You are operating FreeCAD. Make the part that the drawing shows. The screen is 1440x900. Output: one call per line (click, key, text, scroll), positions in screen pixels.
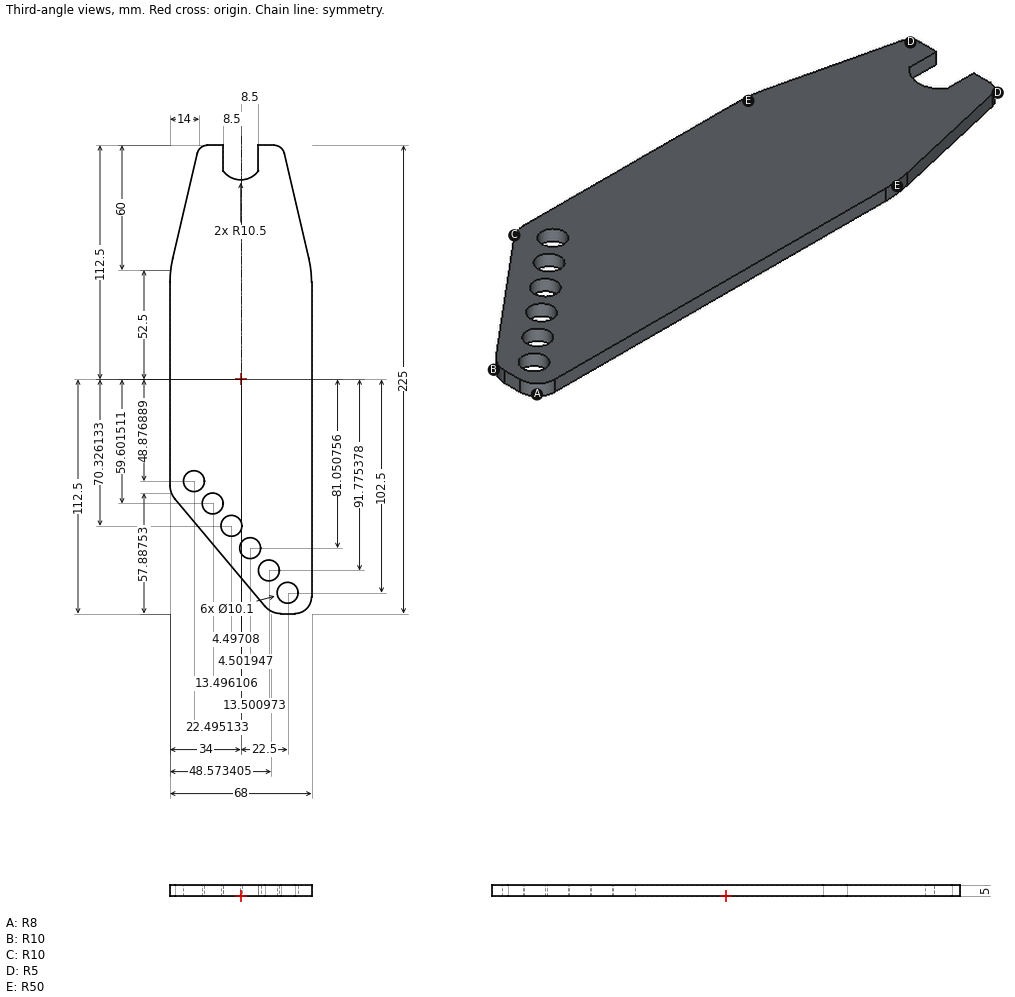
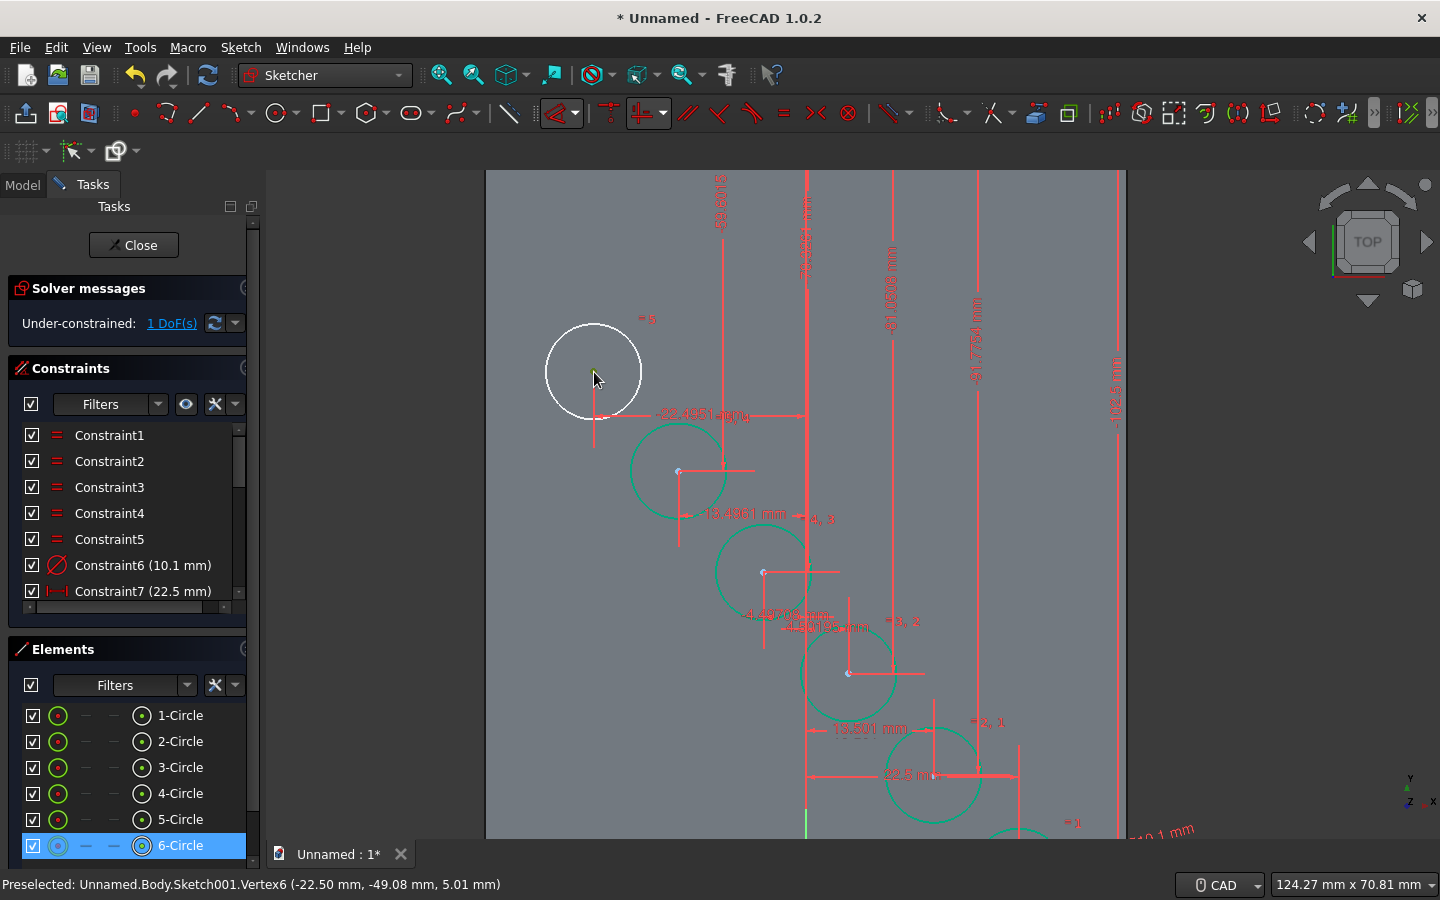
key(i)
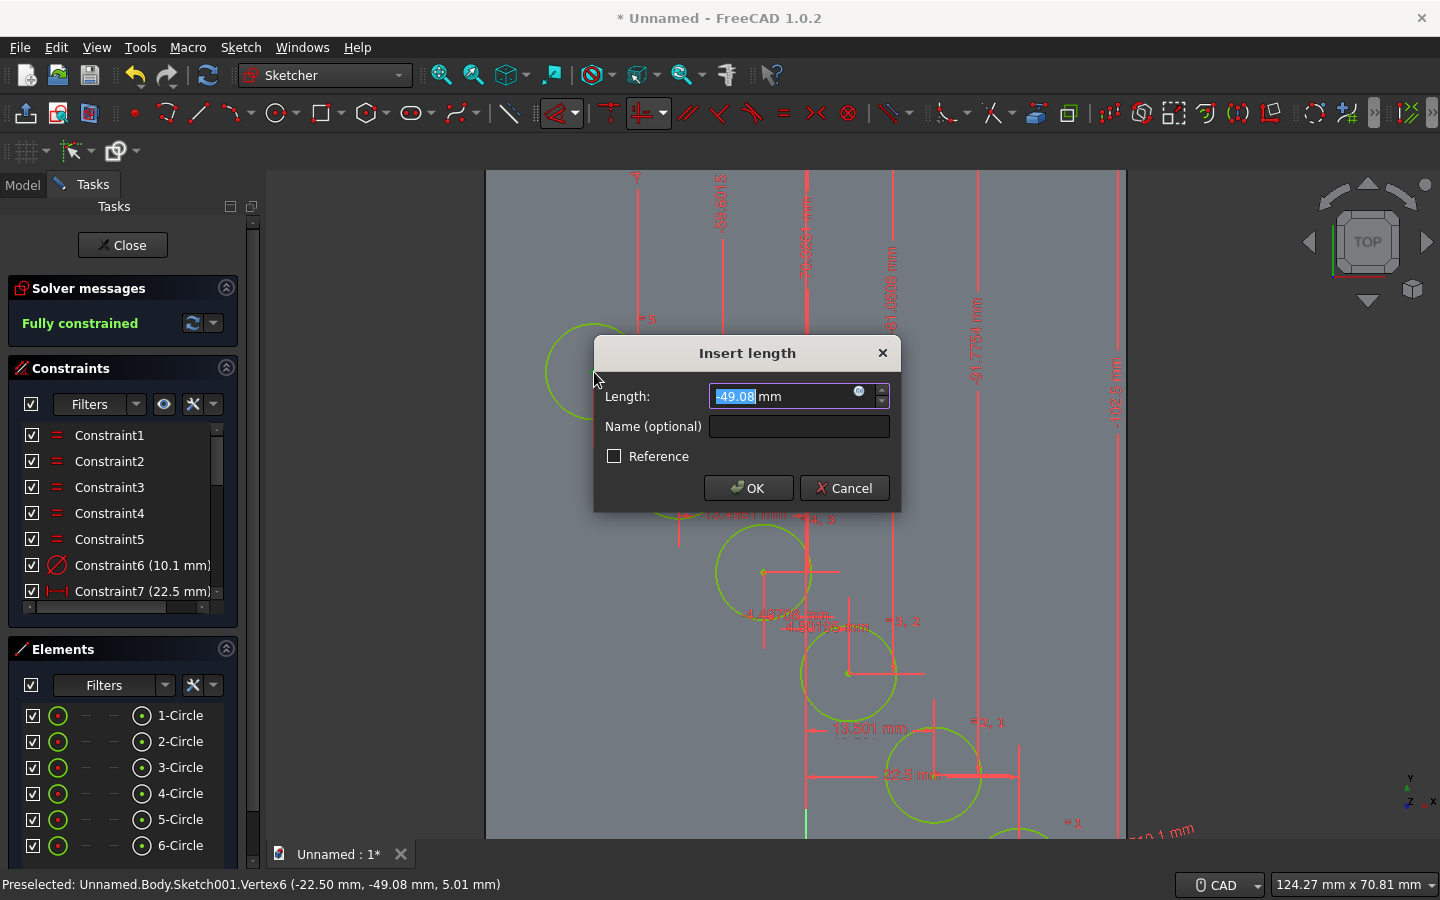
text(-48.876889)
key(Return)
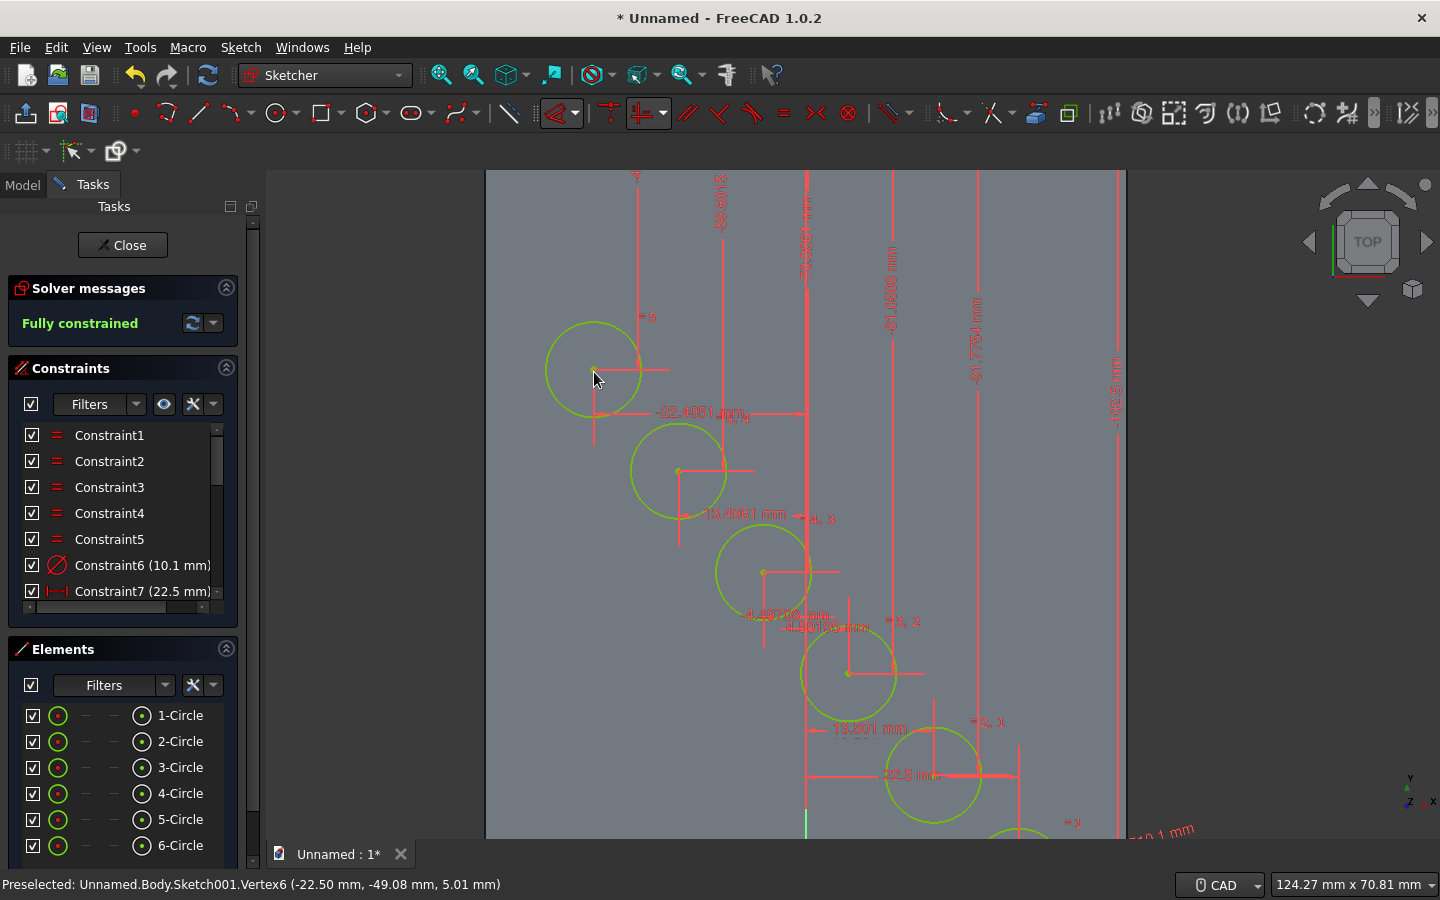
click(123, 245)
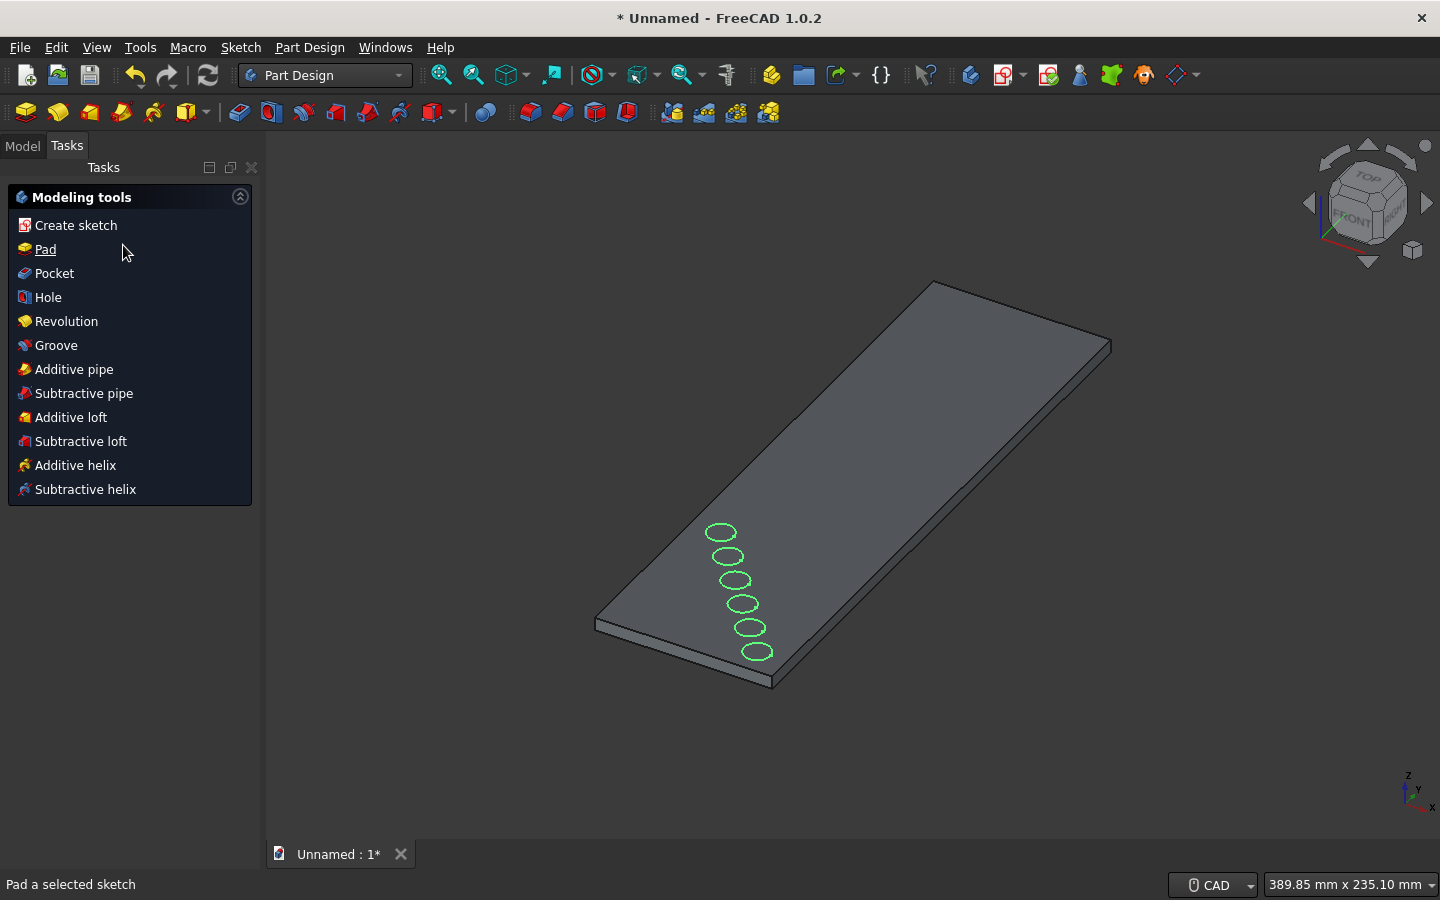
click(240, 112)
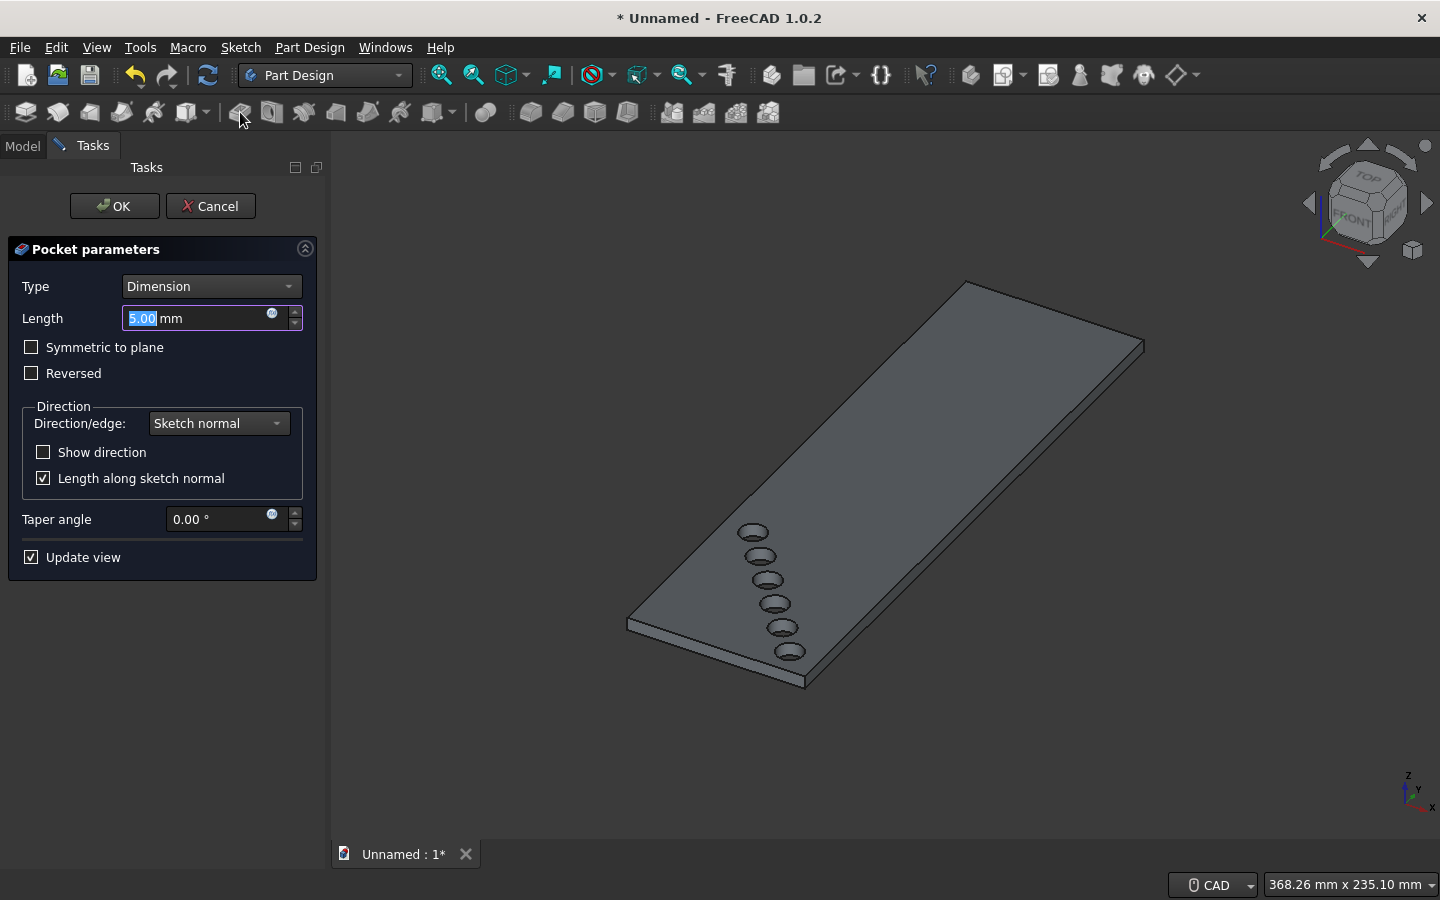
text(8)
key(Tab)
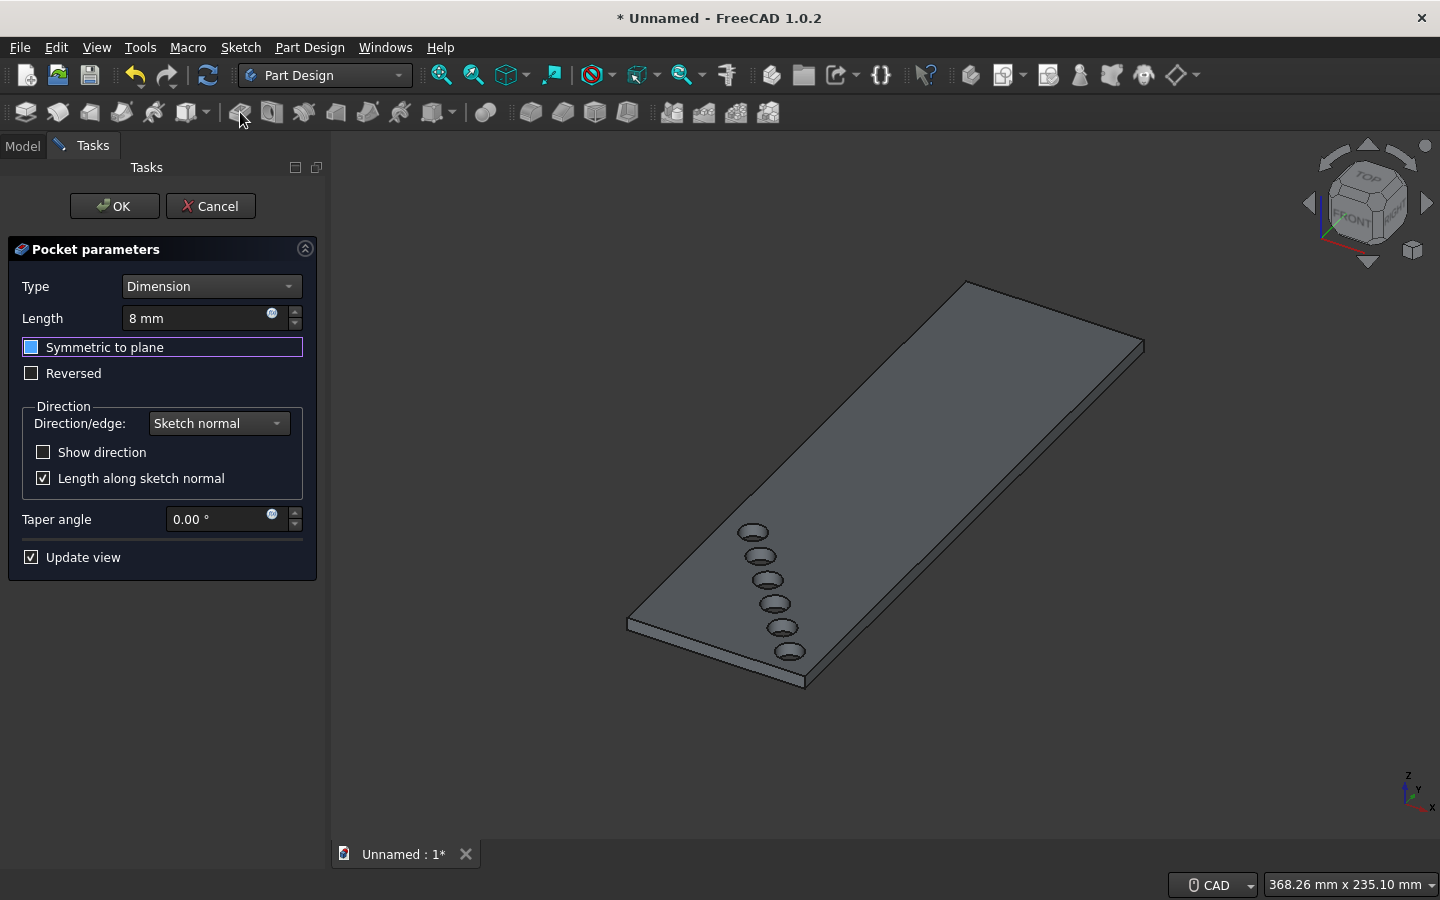
click(115, 206)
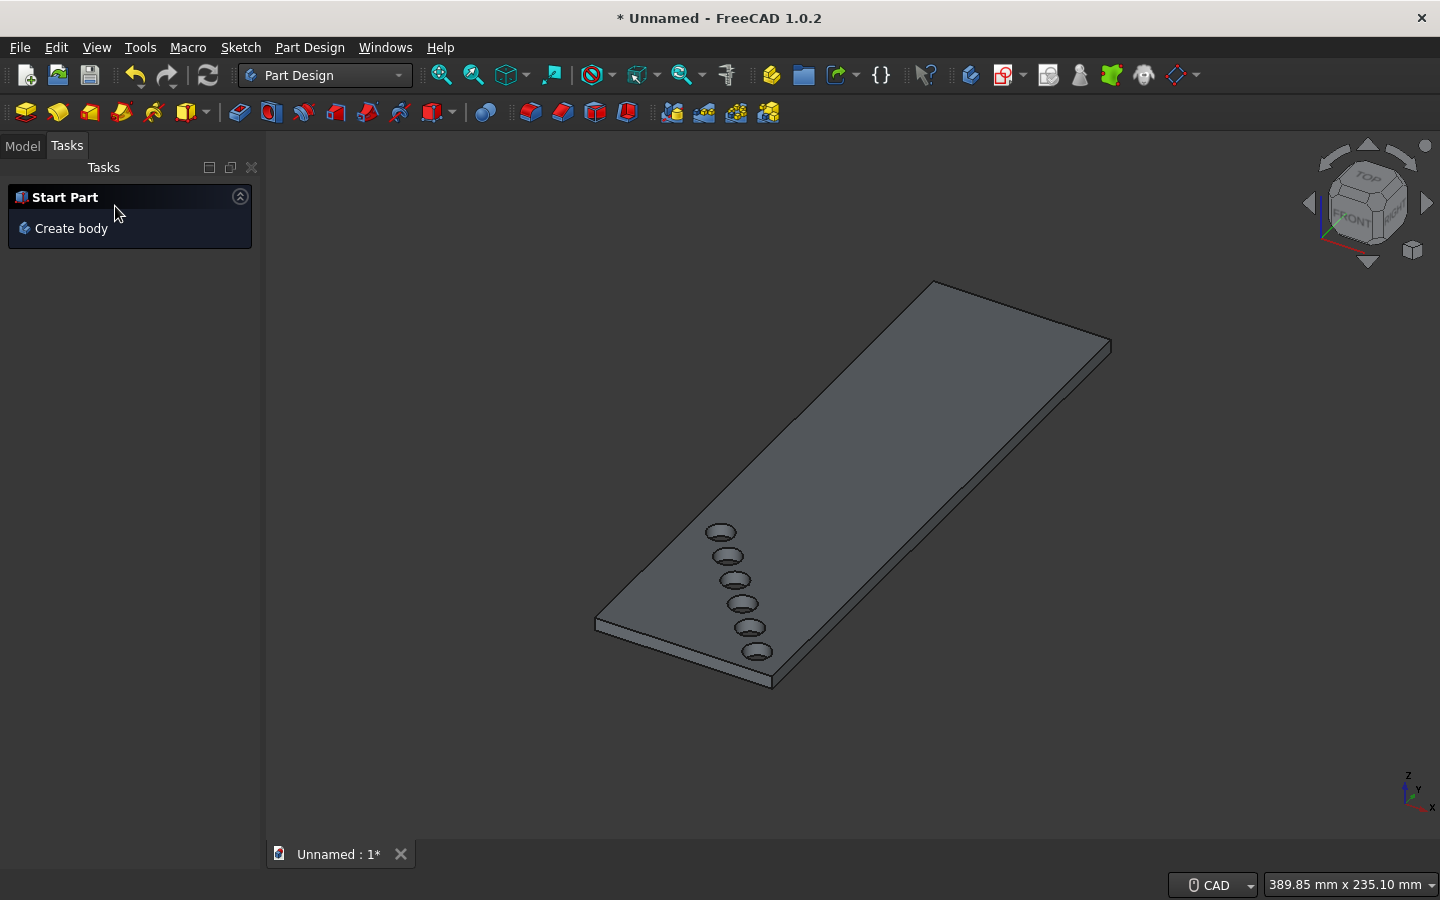
click(772, 682)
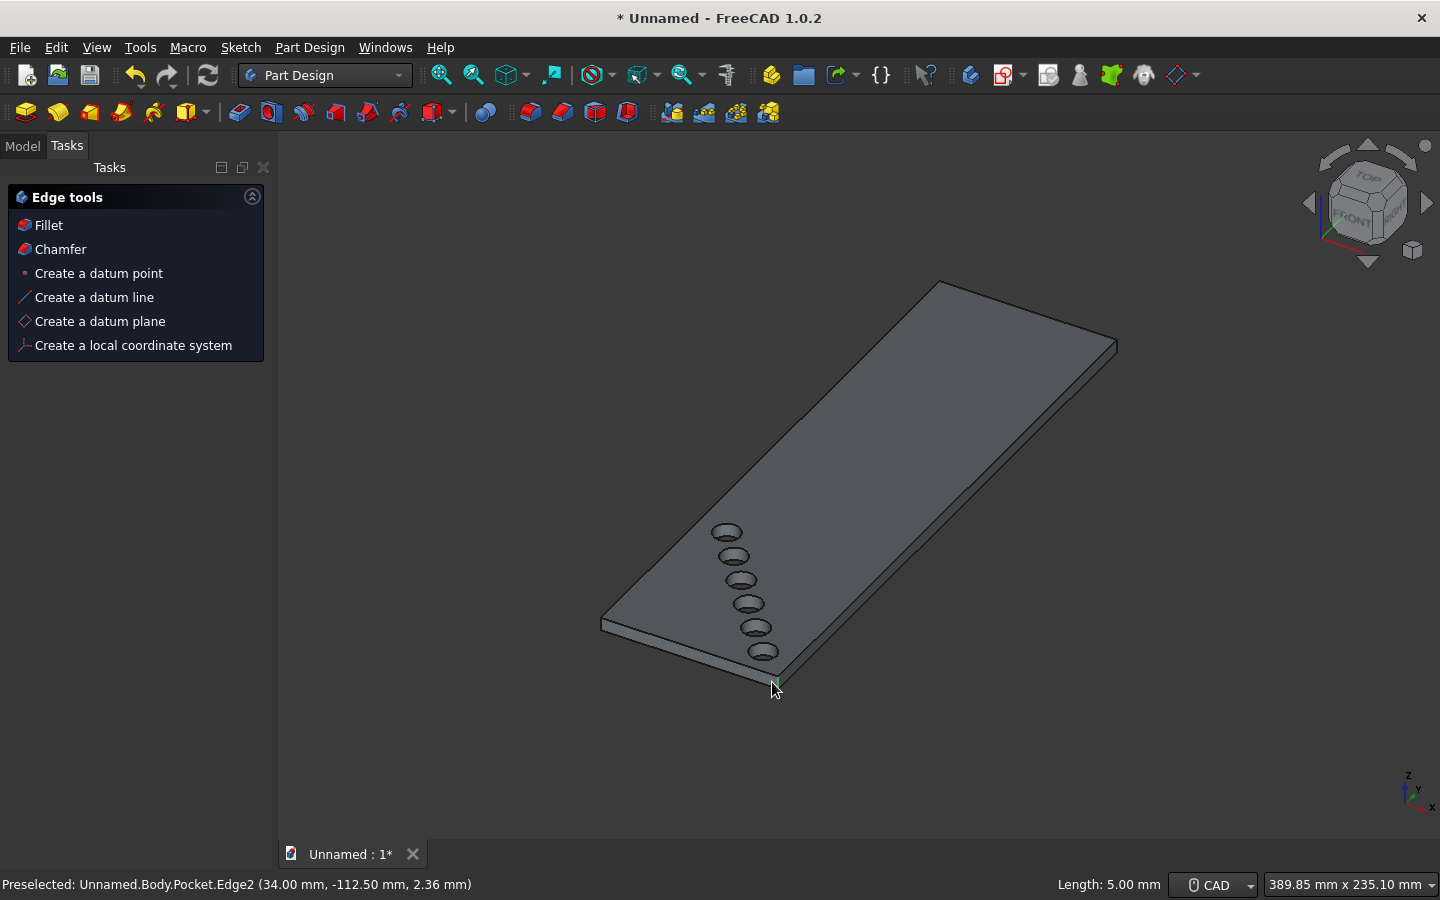
click(532, 112)